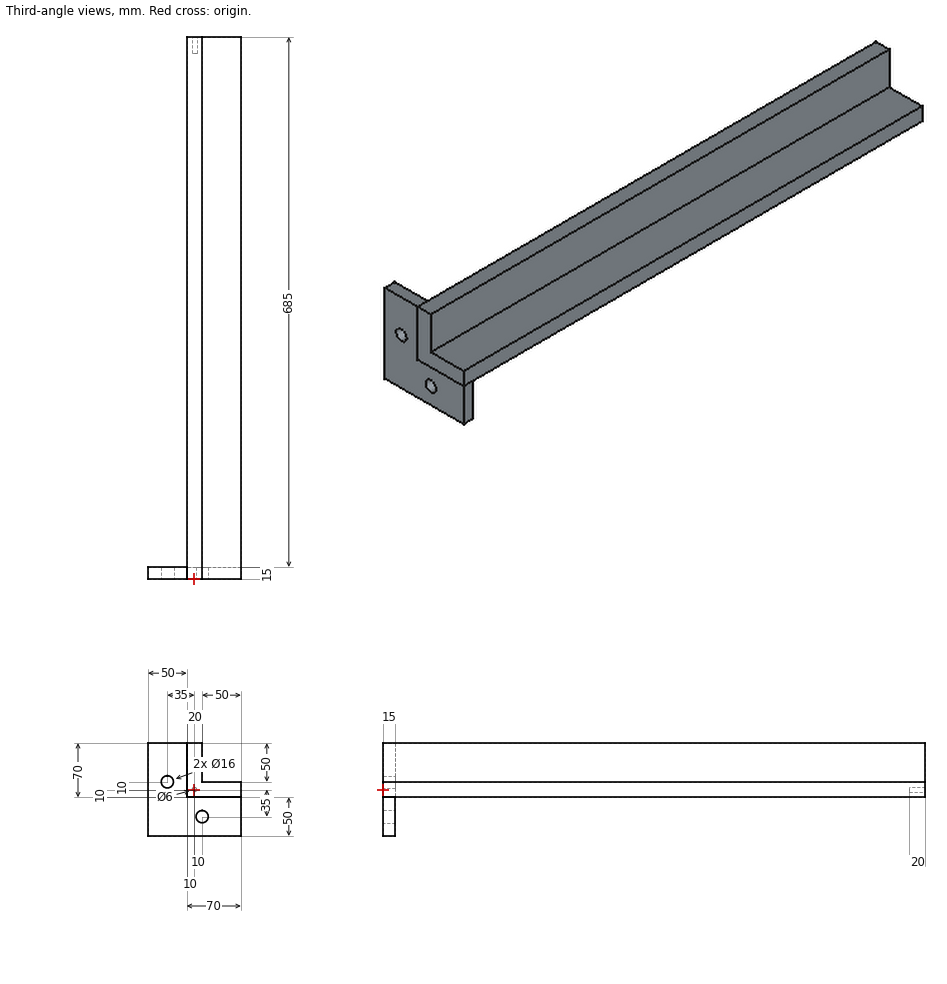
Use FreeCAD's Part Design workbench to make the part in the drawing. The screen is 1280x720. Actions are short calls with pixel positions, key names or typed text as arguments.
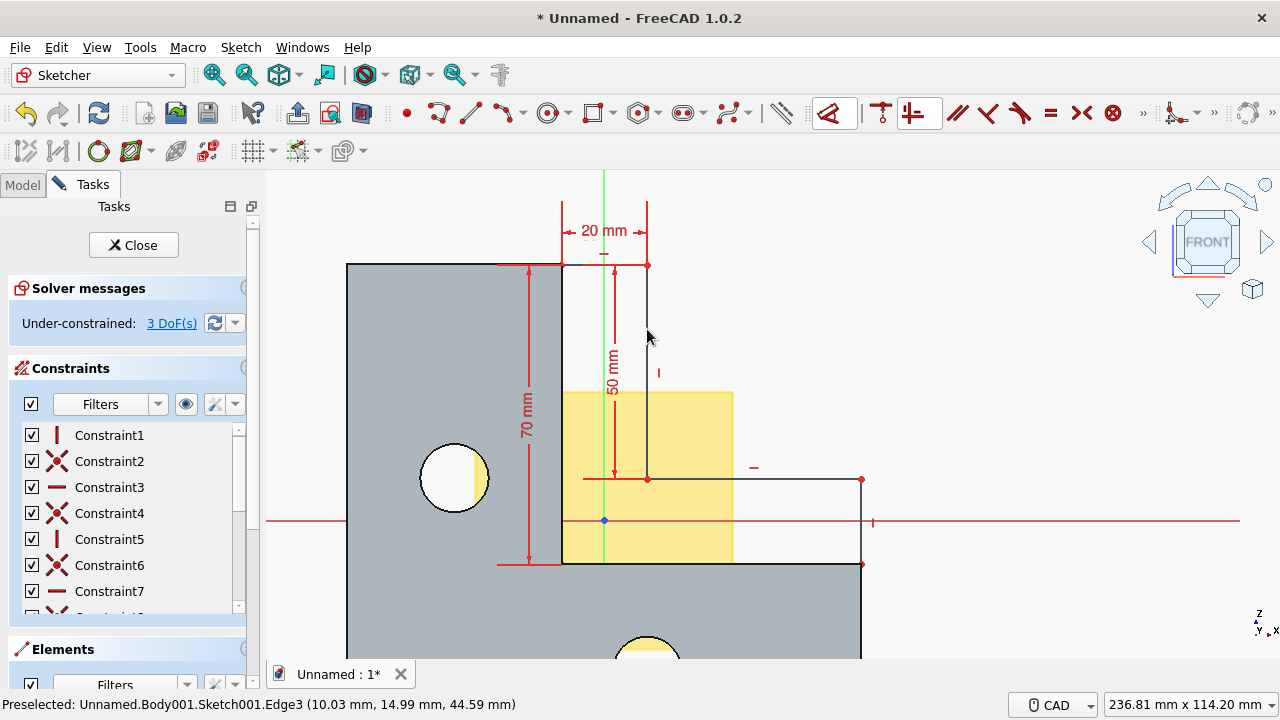
click(711, 479)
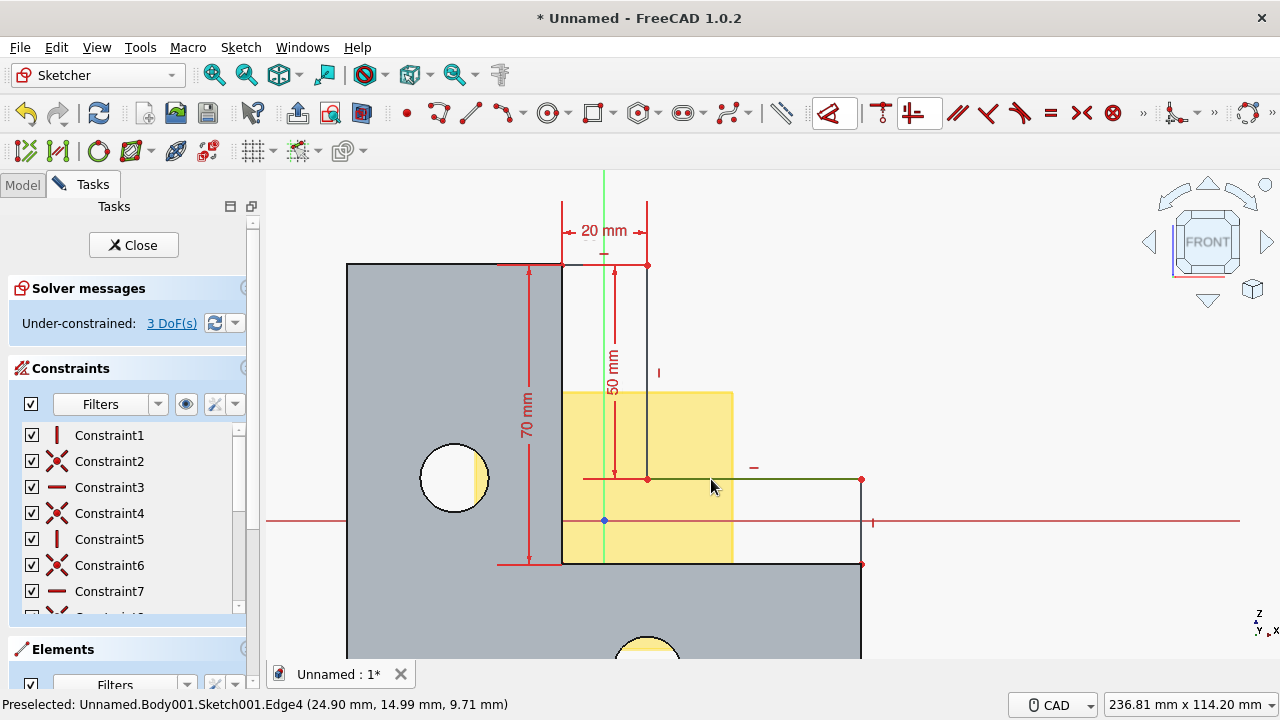
click(852, 114)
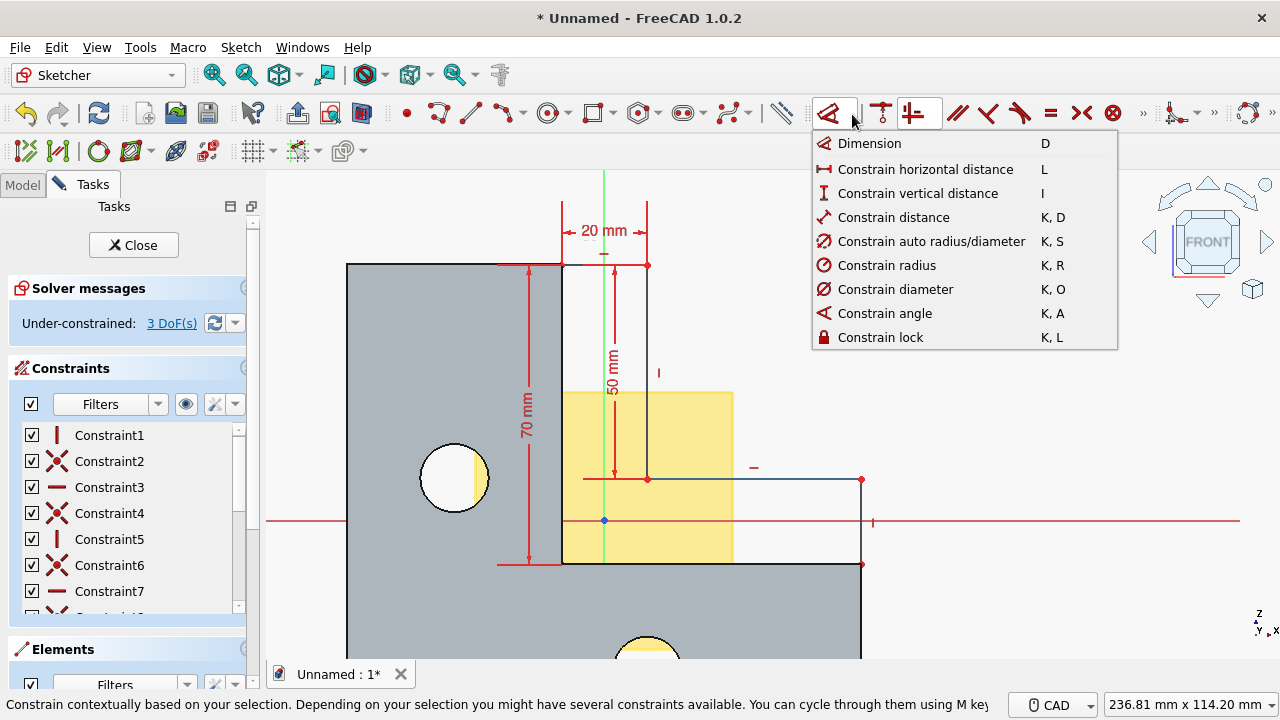
click(965, 169)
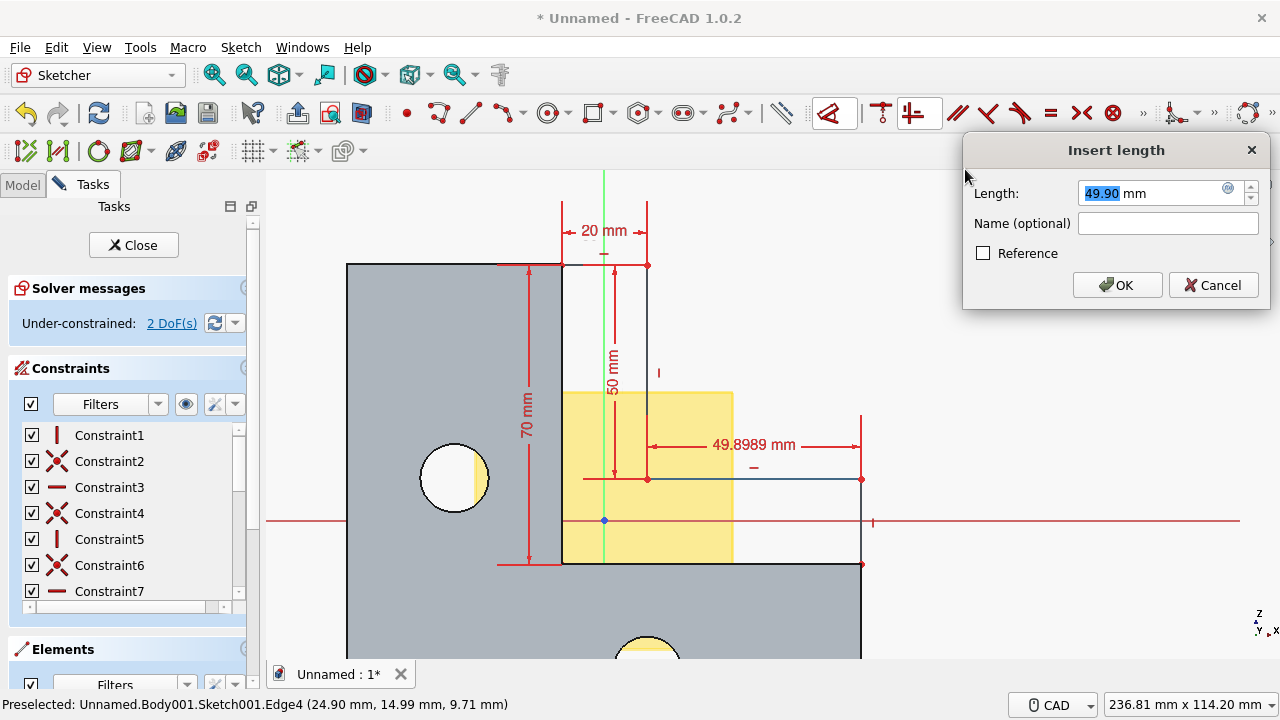
text(50)
key(Return)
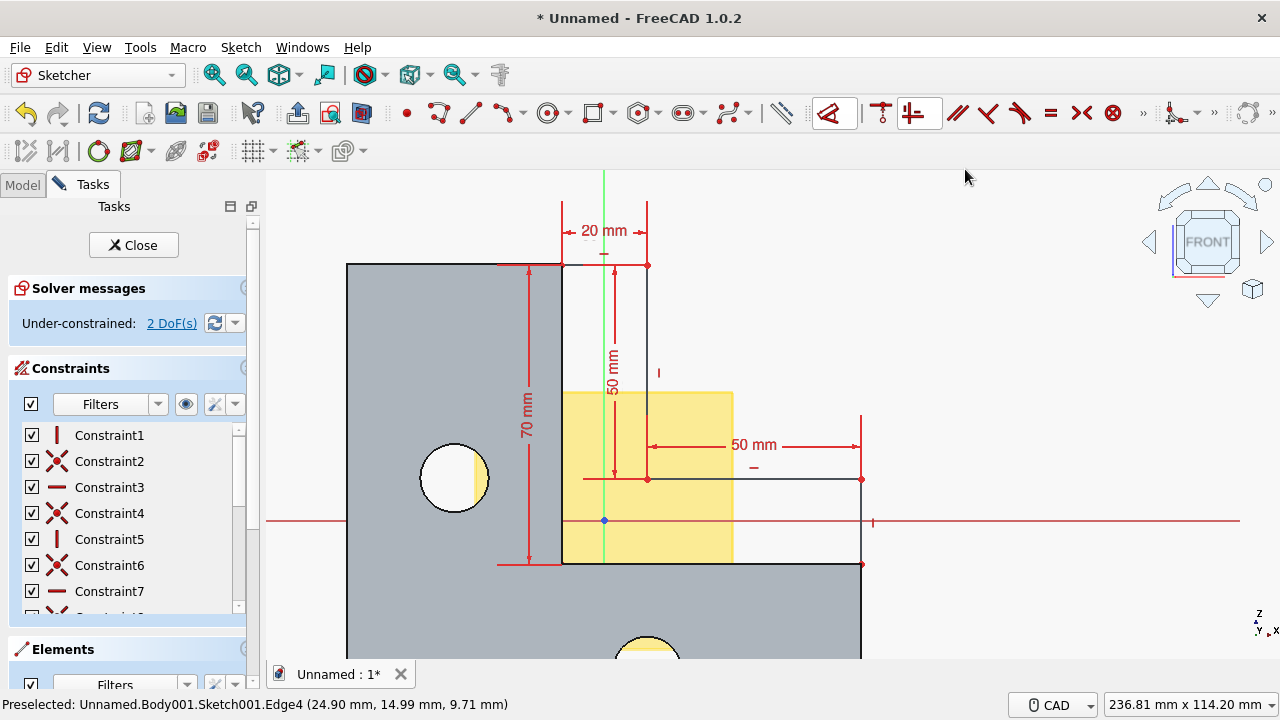
click(562, 565)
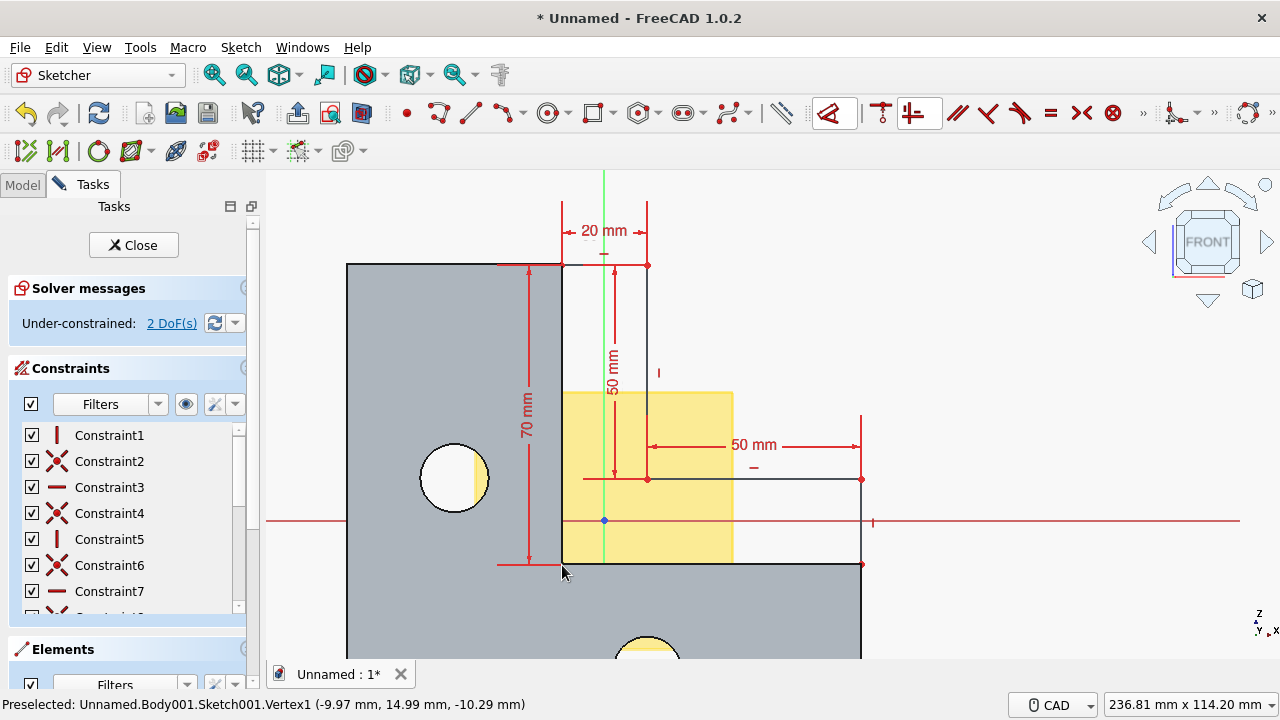
click(852, 114)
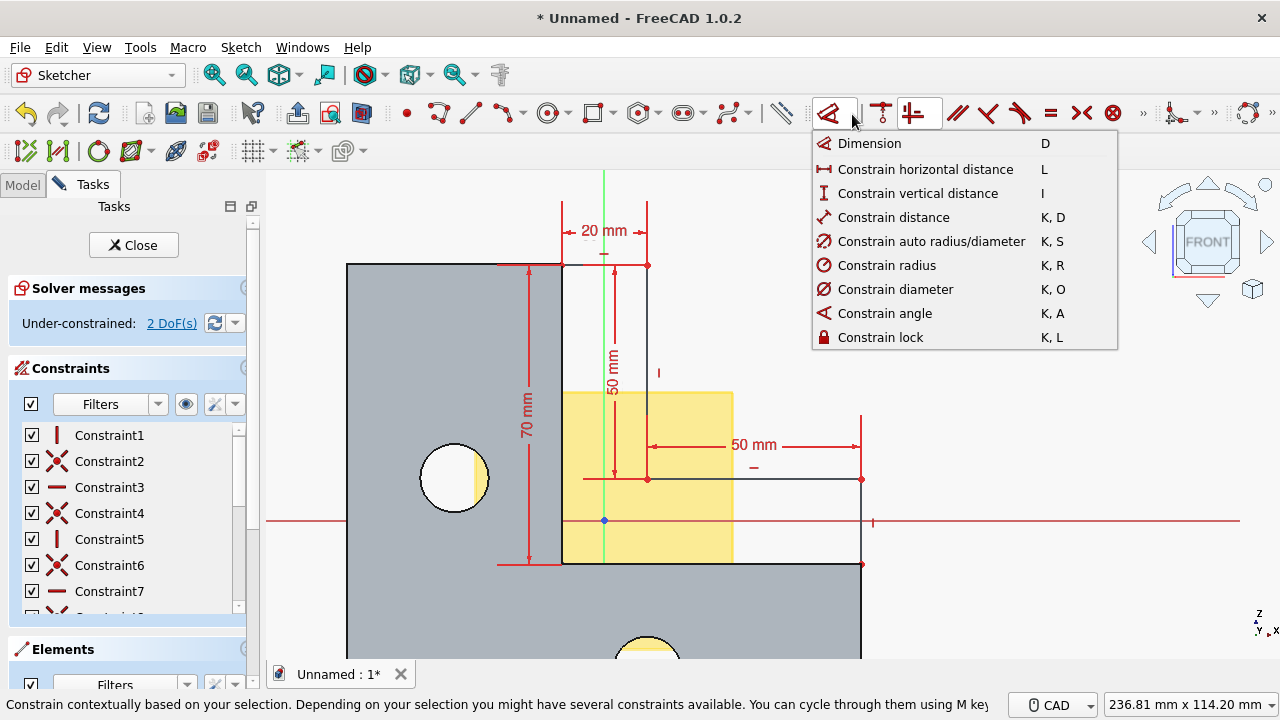
click(965, 169)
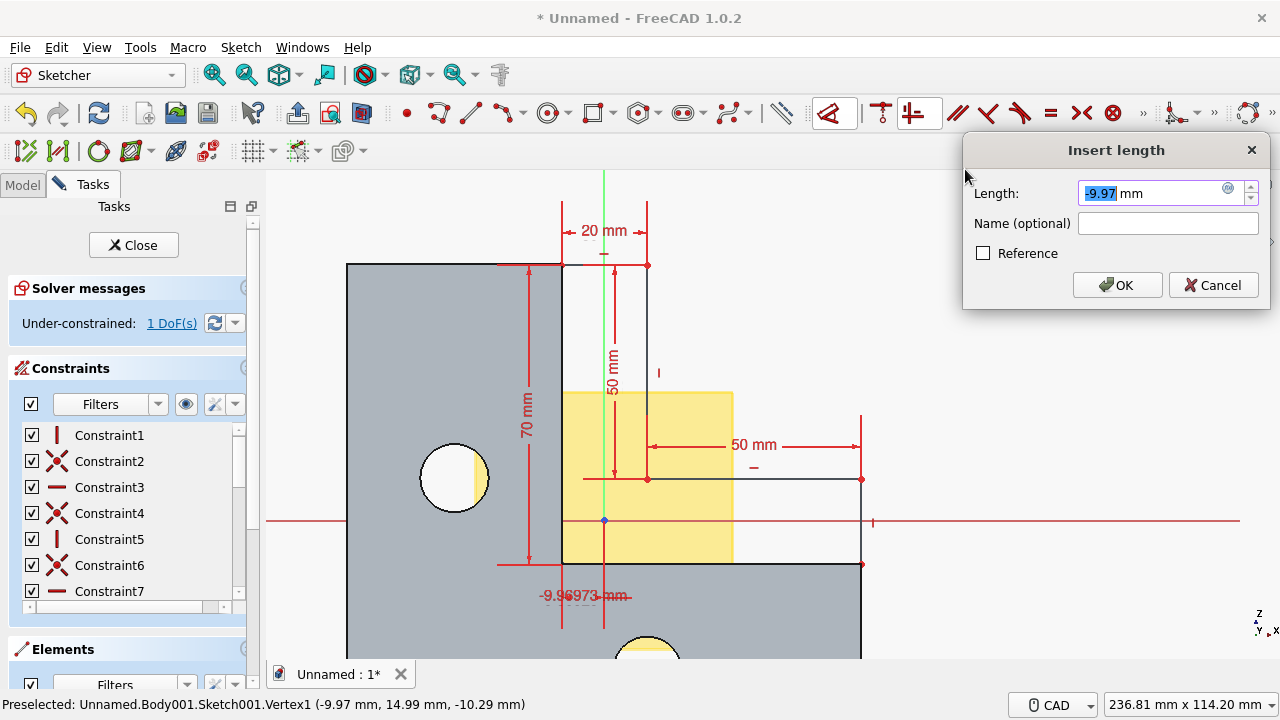
text(-10)
key(Return)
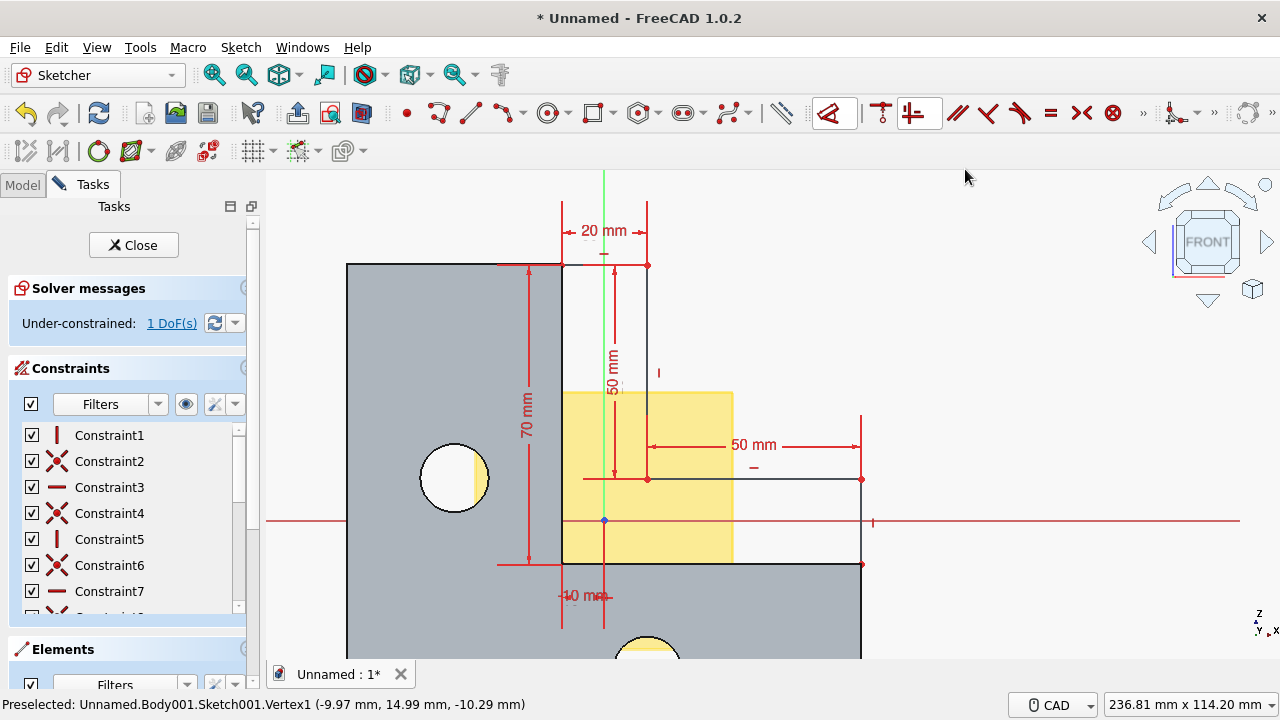
click(562, 565)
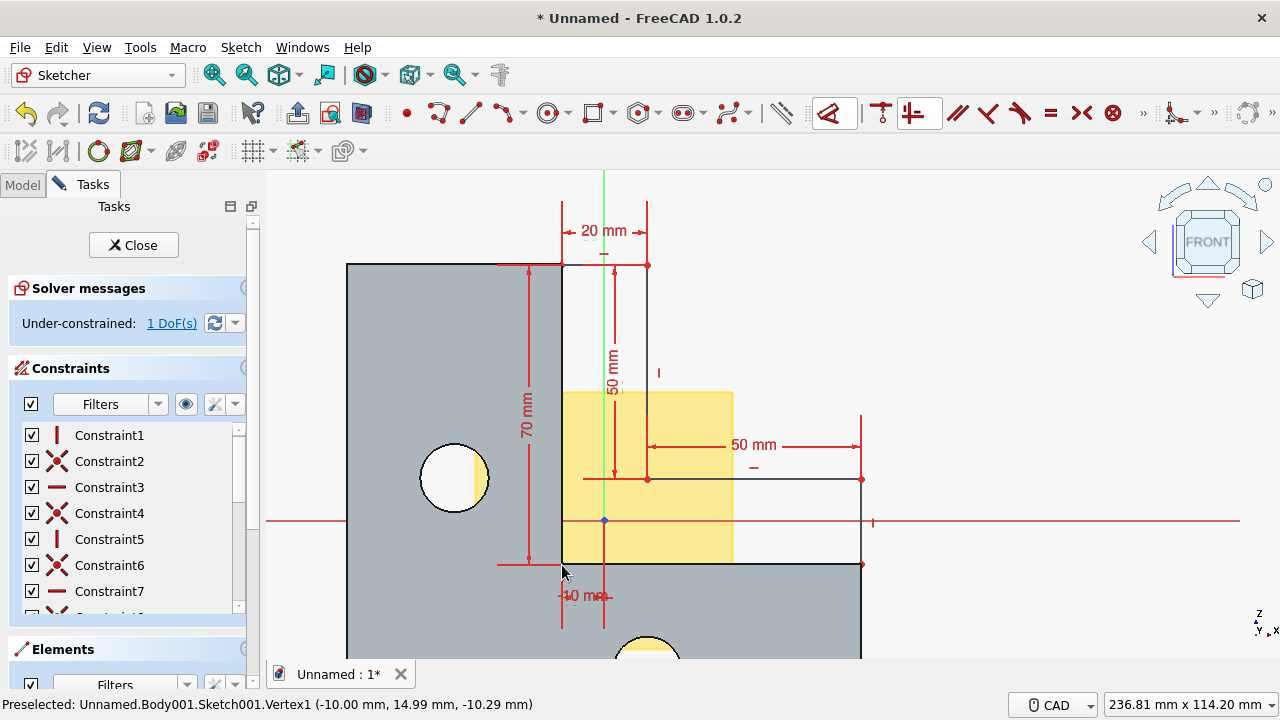
click(852, 114)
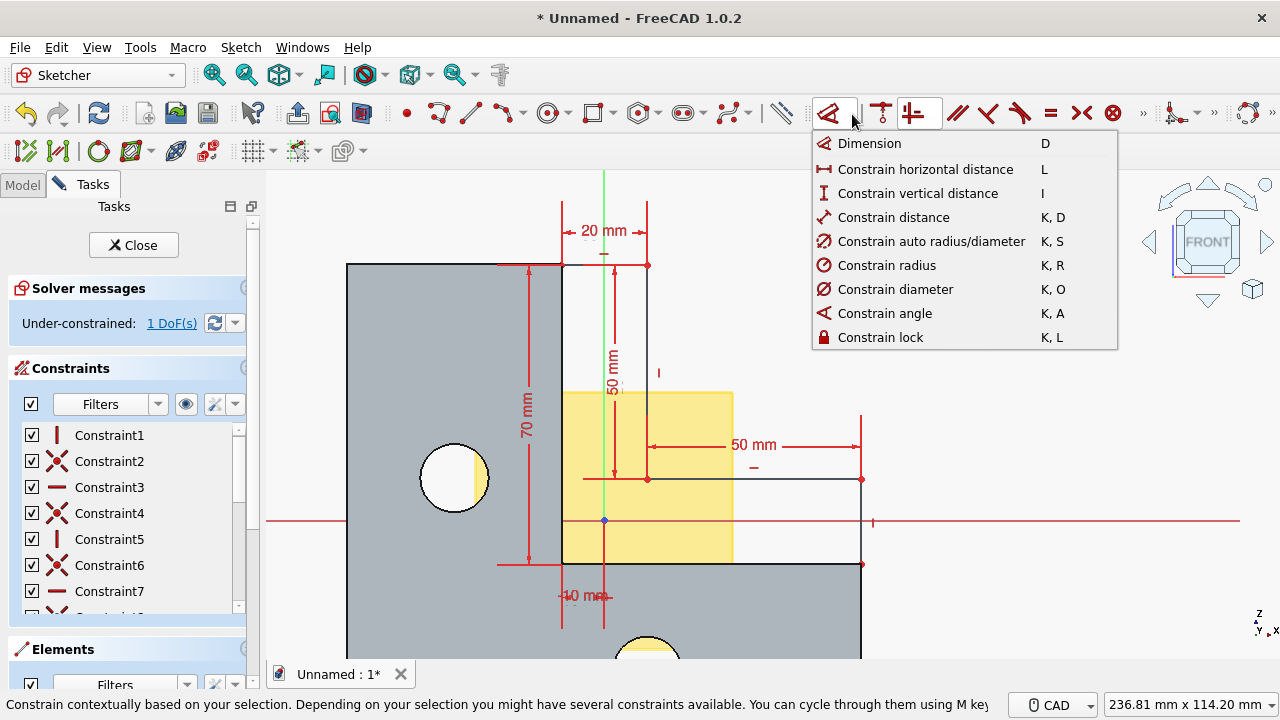
click(965, 193)